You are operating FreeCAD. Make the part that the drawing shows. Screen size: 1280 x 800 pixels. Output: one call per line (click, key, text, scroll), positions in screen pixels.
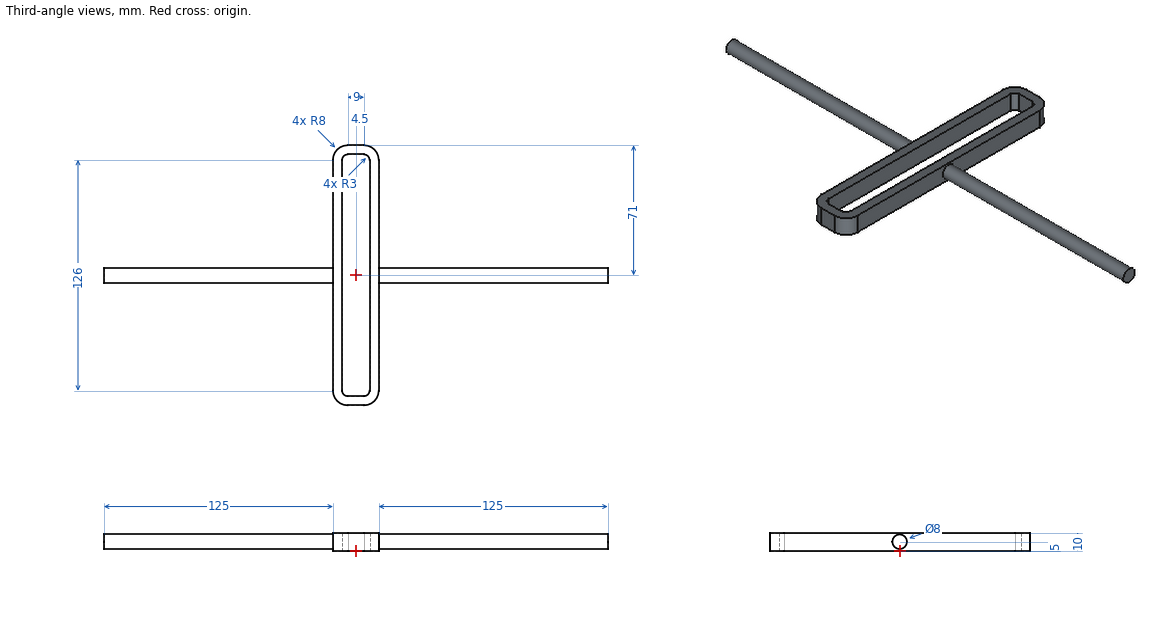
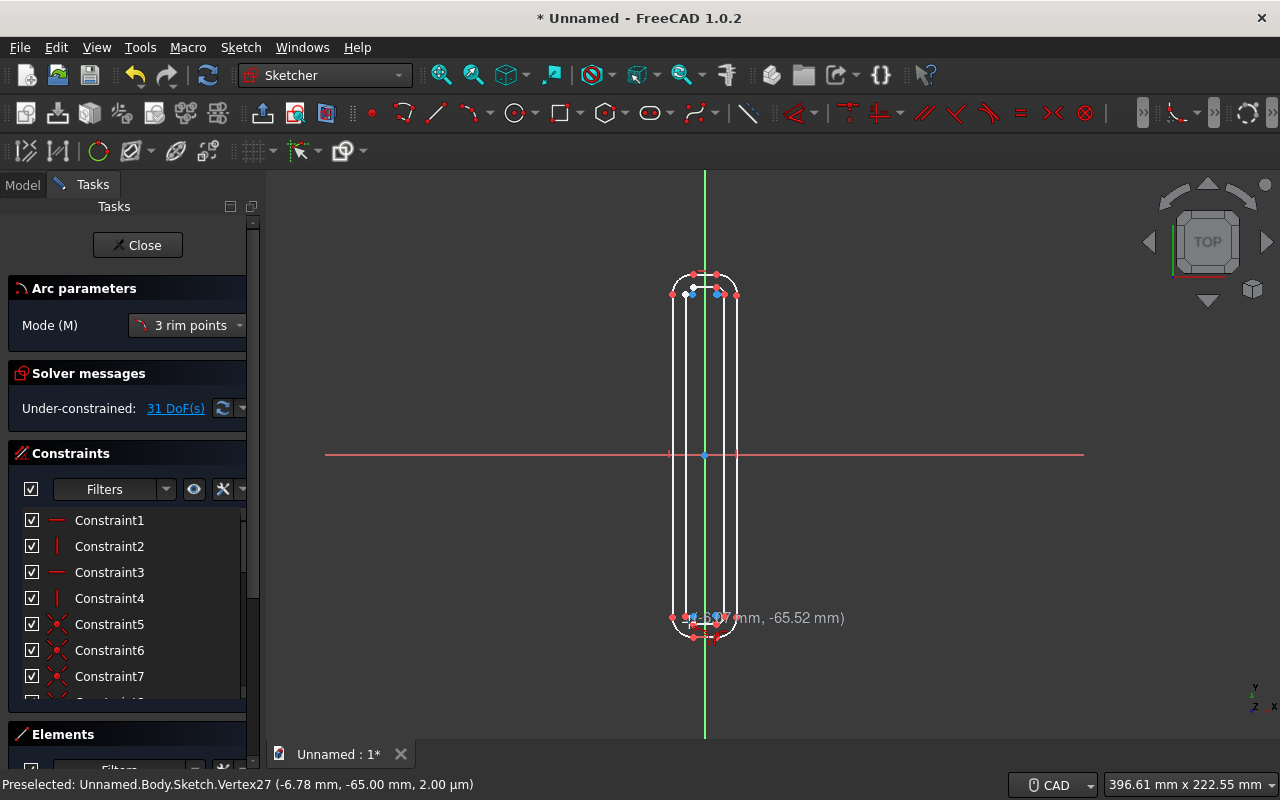
scroll(686, 294, up, 4)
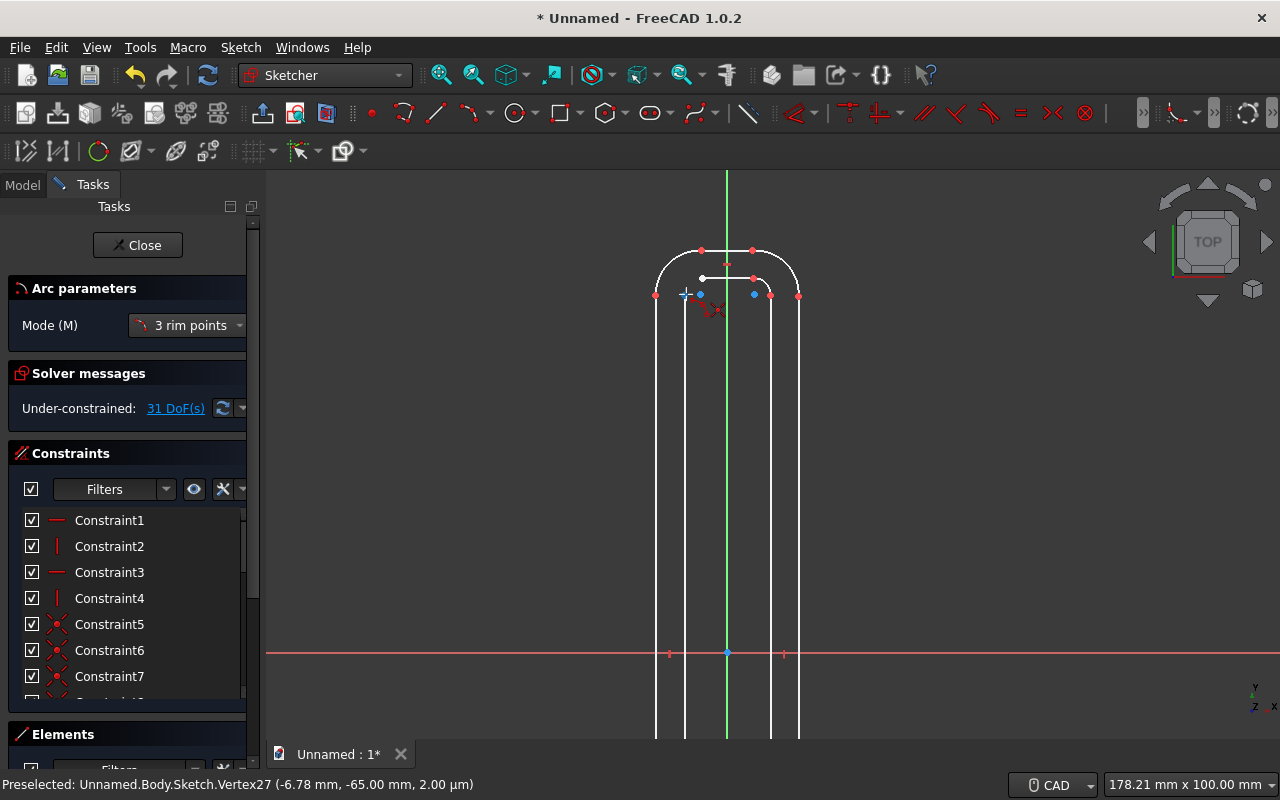
click(685, 295)
click(702, 278)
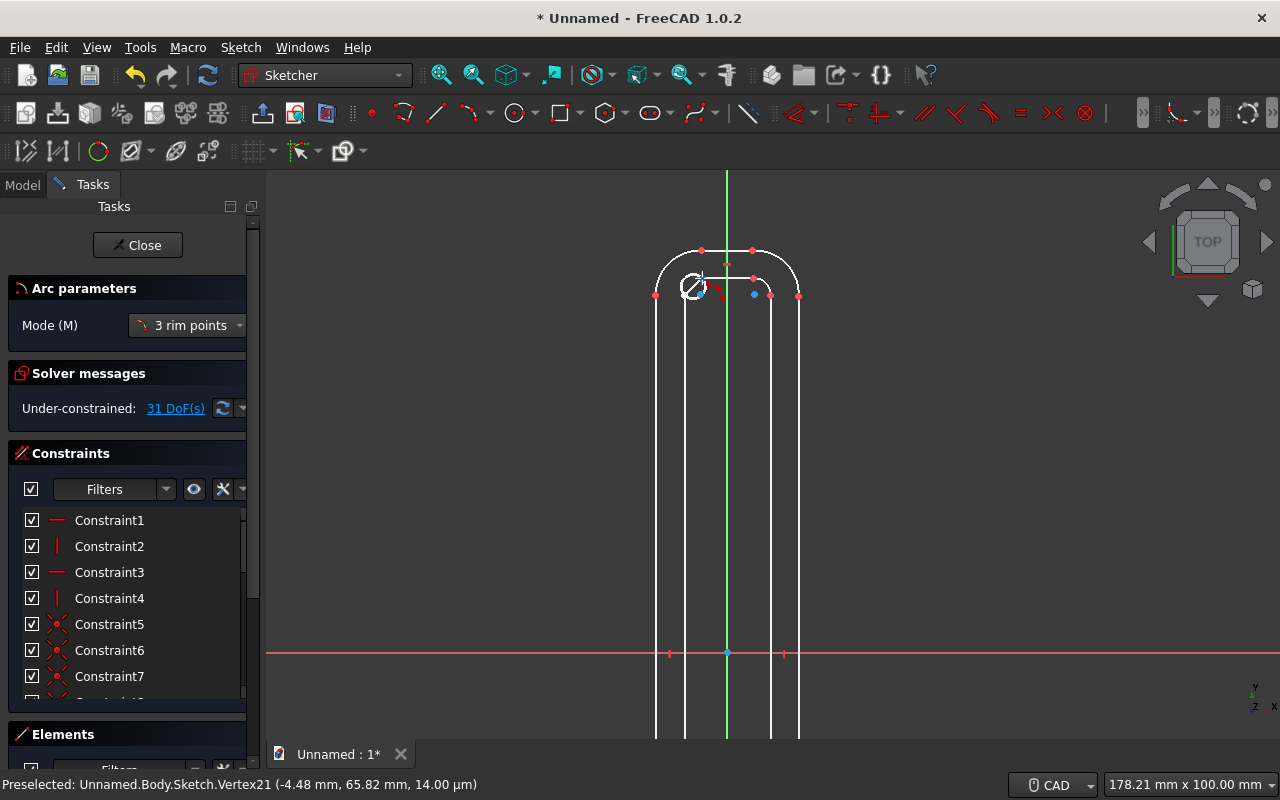
scroll(690, 282, up, 6)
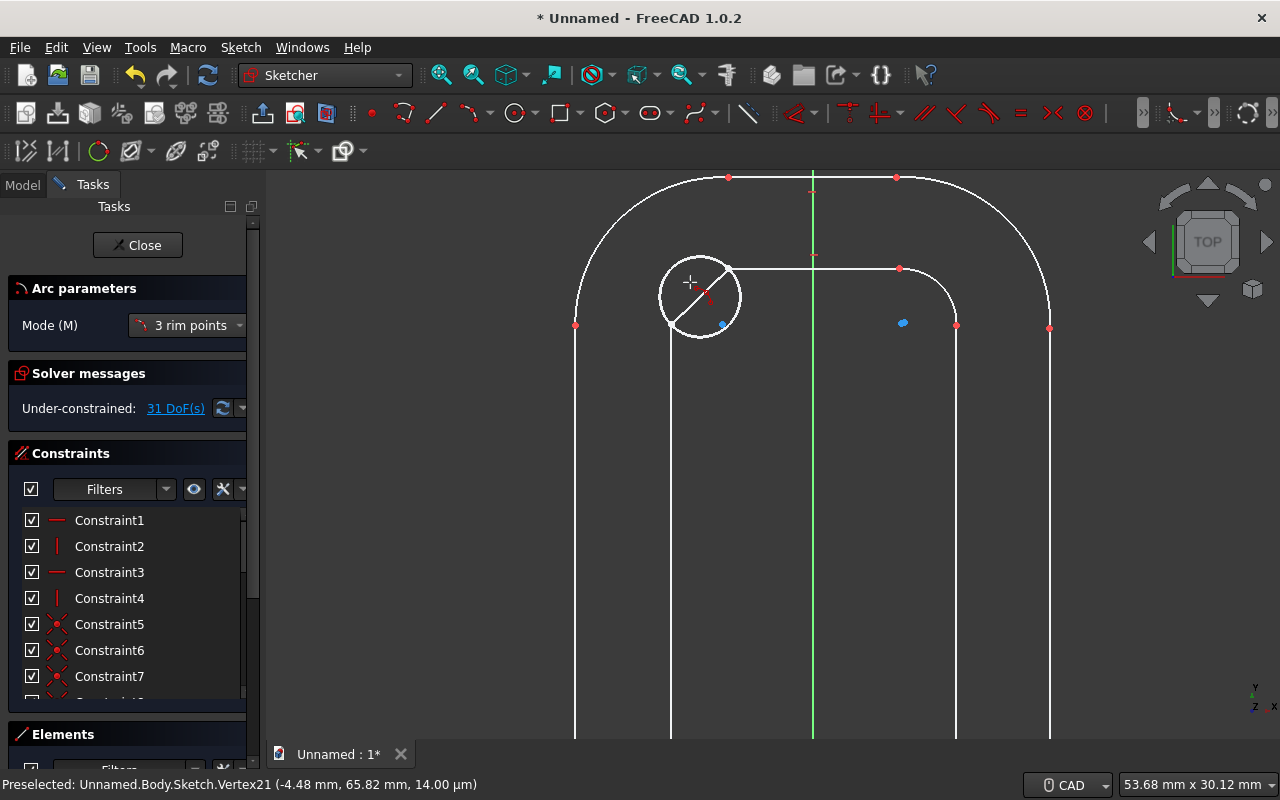
click(688, 282)
key(Escape)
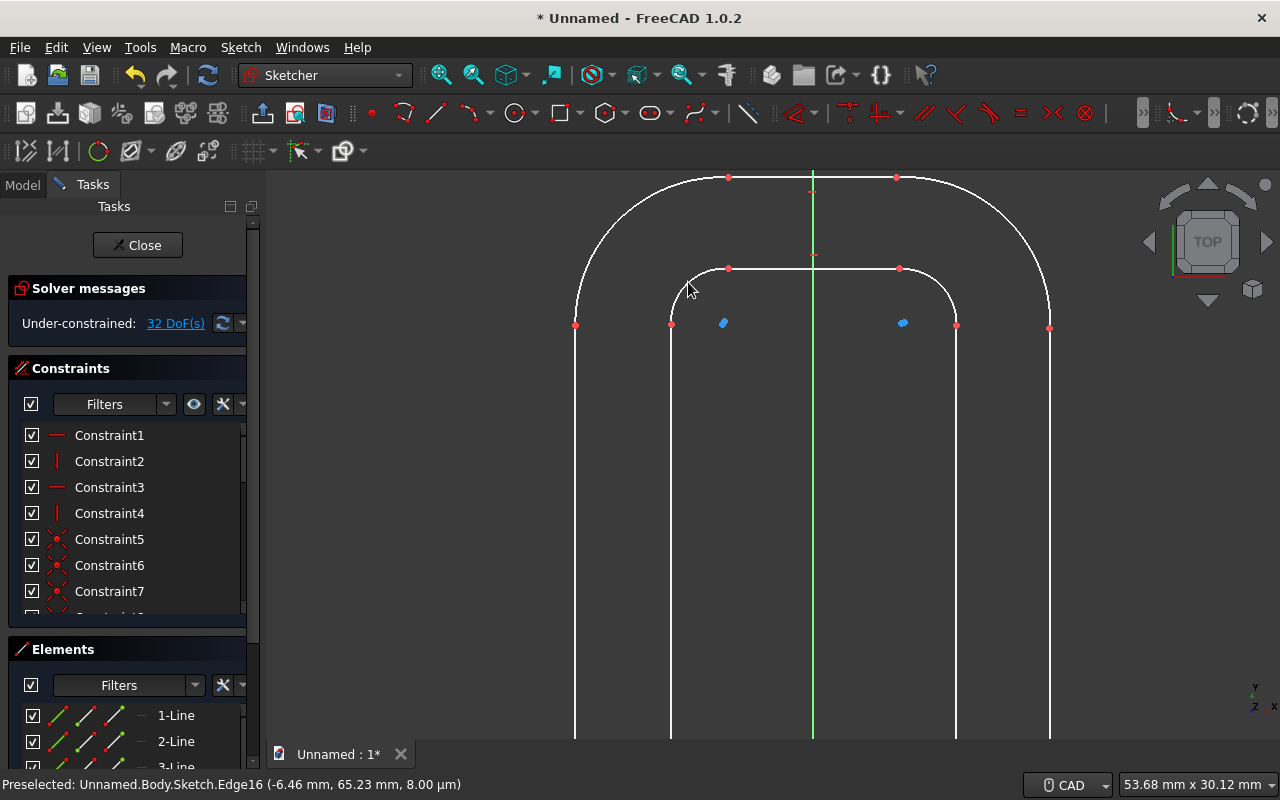
scroll(687, 289, down, 10)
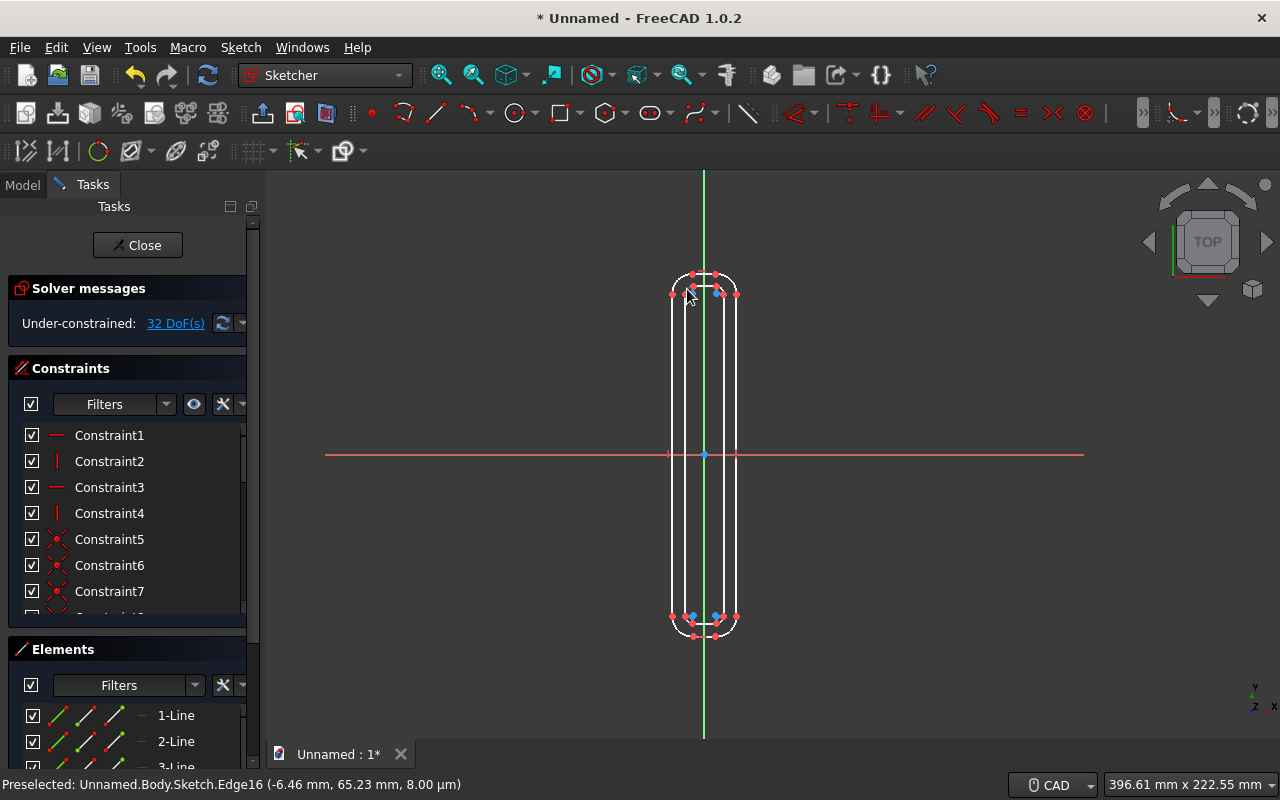
scroll(709, 274, up, 6)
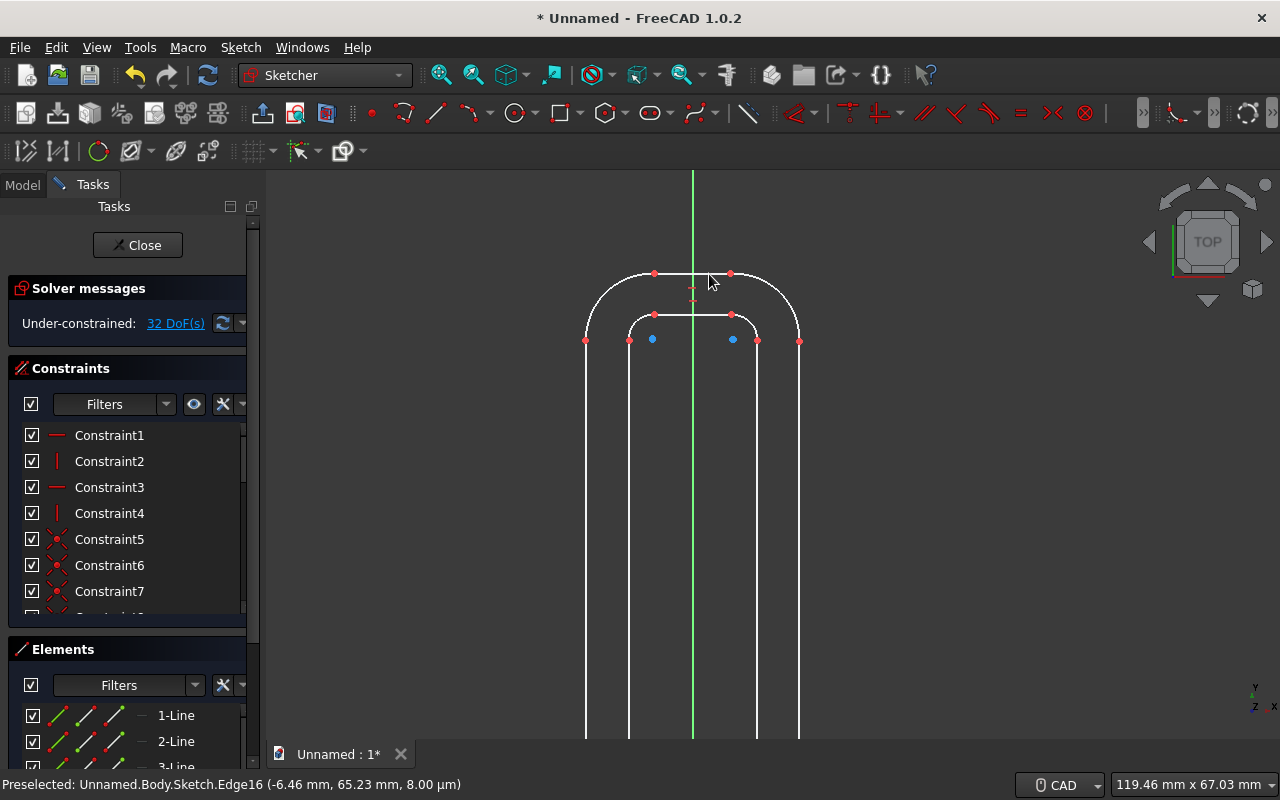
click(707, 274)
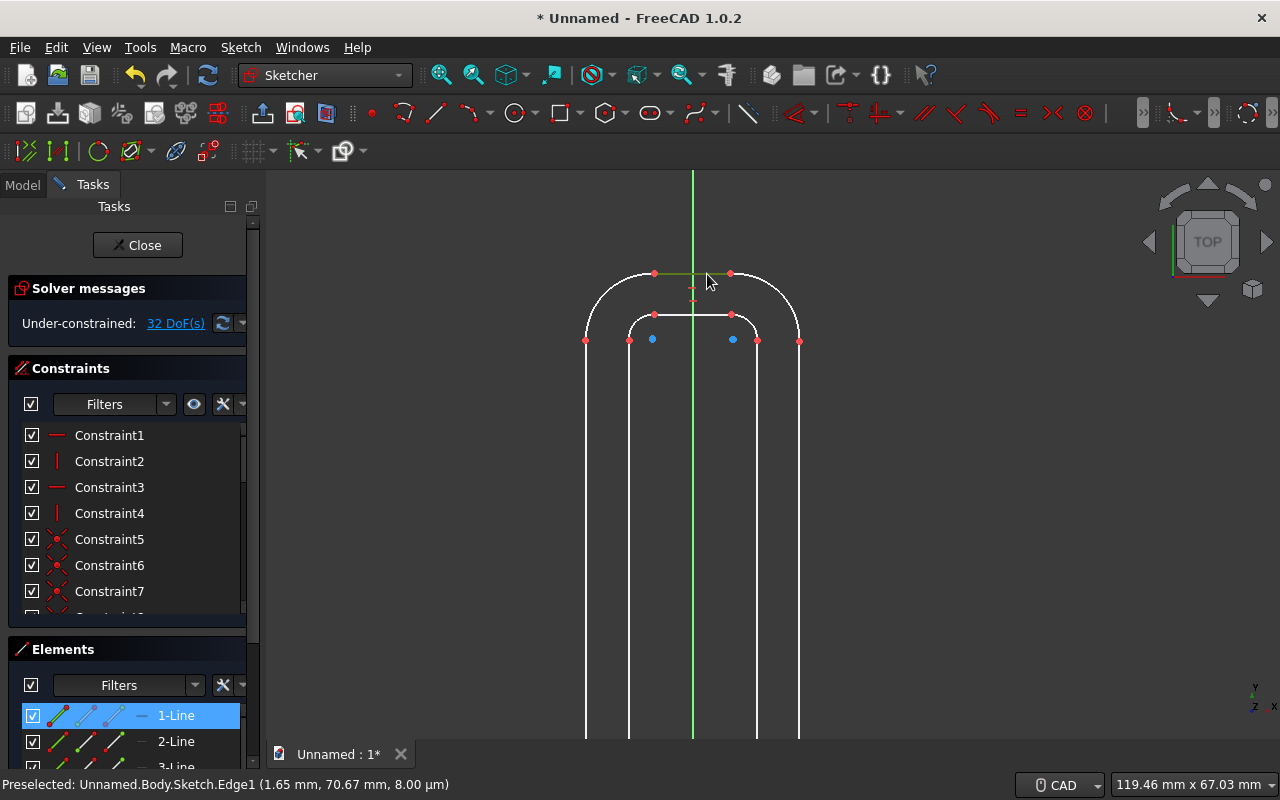
click(624, 280)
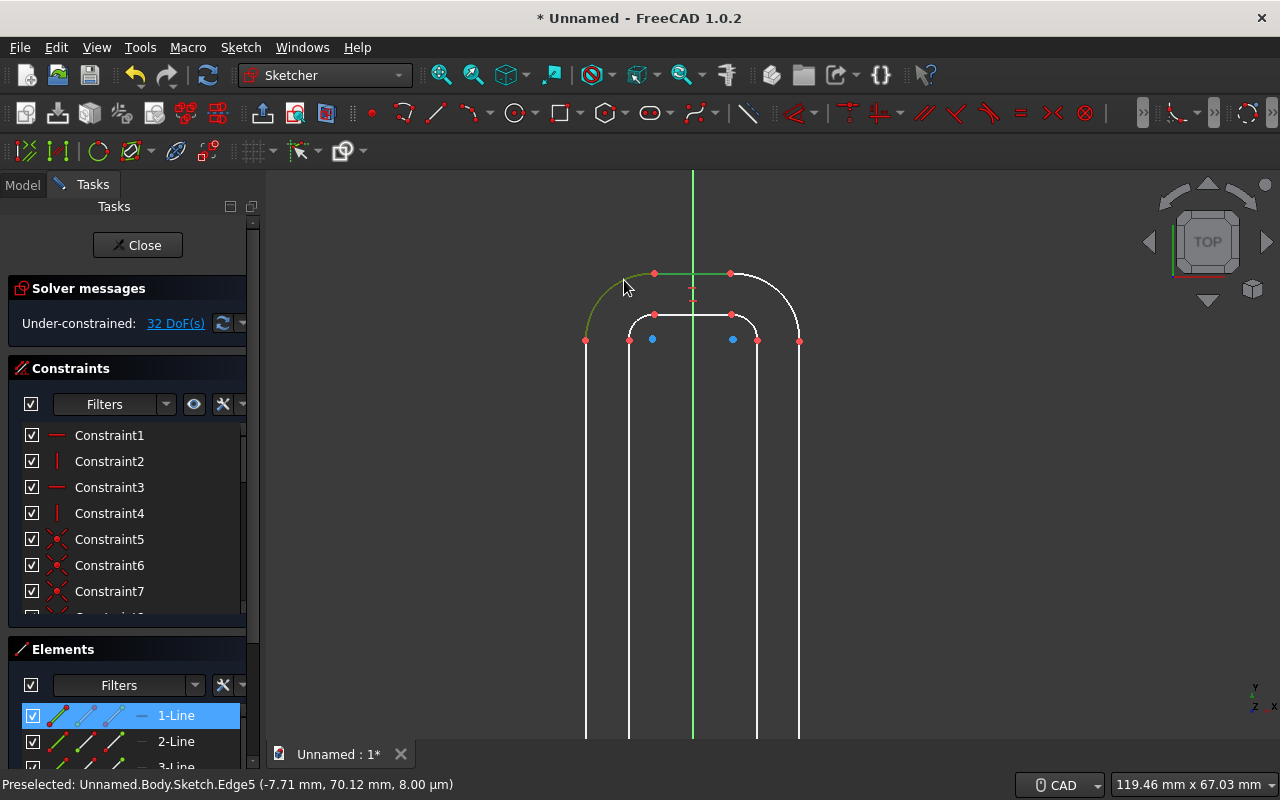
click(990, 114)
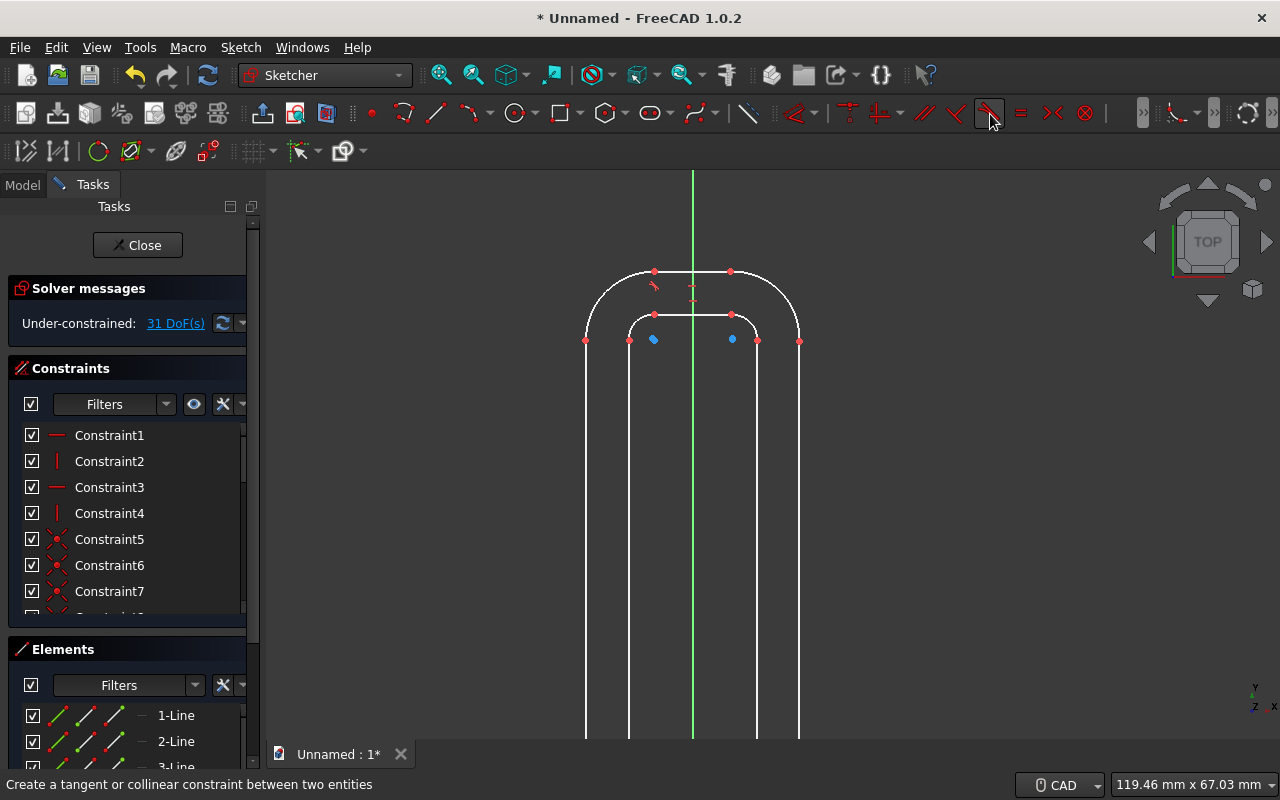
click(707, 272)